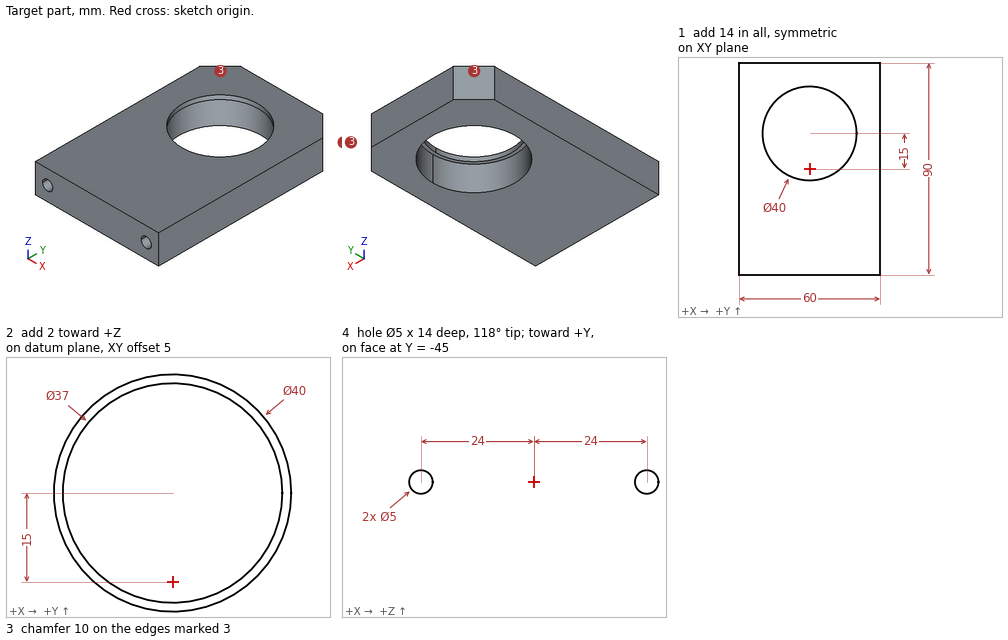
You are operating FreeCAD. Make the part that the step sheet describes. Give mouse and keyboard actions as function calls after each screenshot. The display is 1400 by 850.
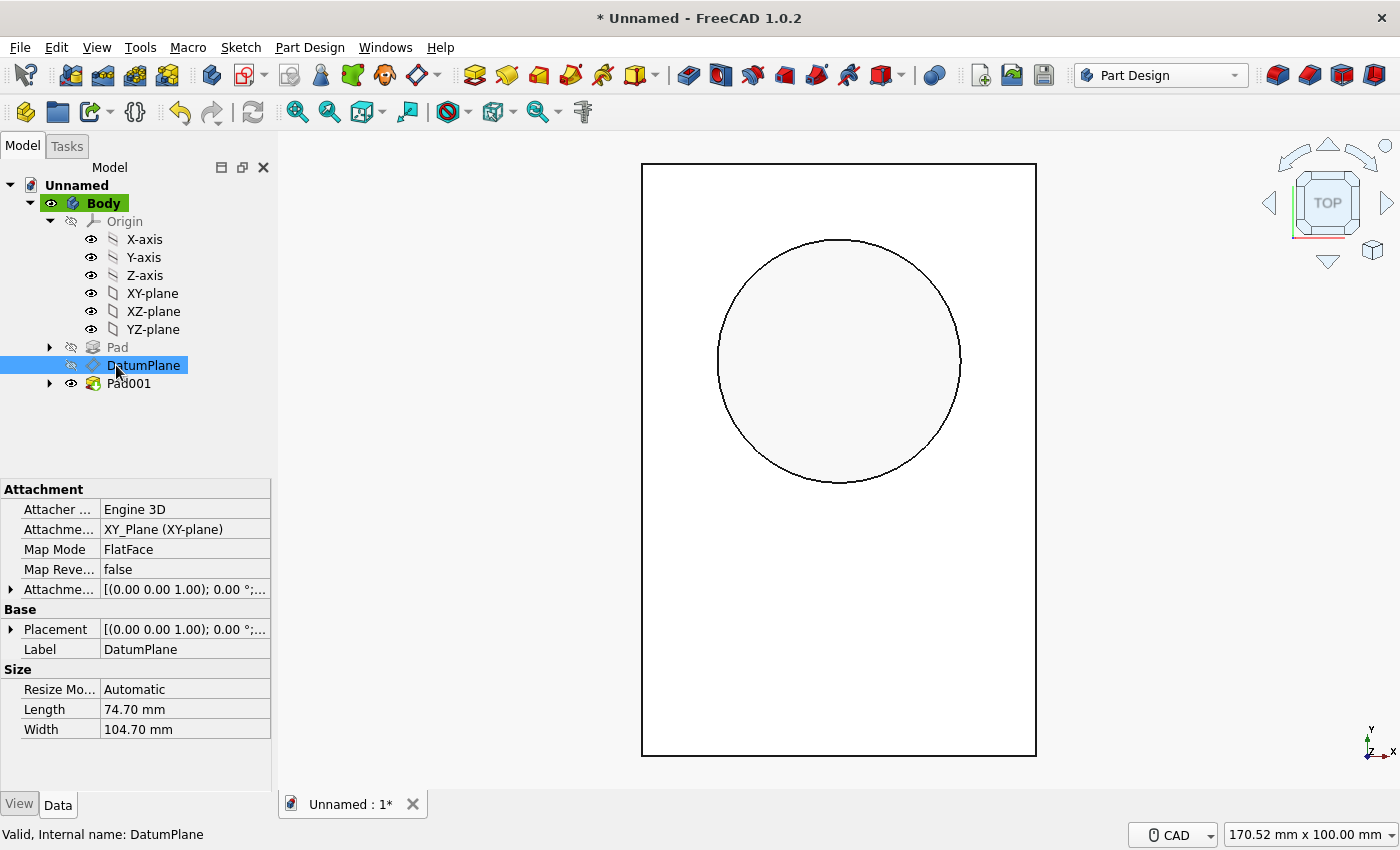
key(1)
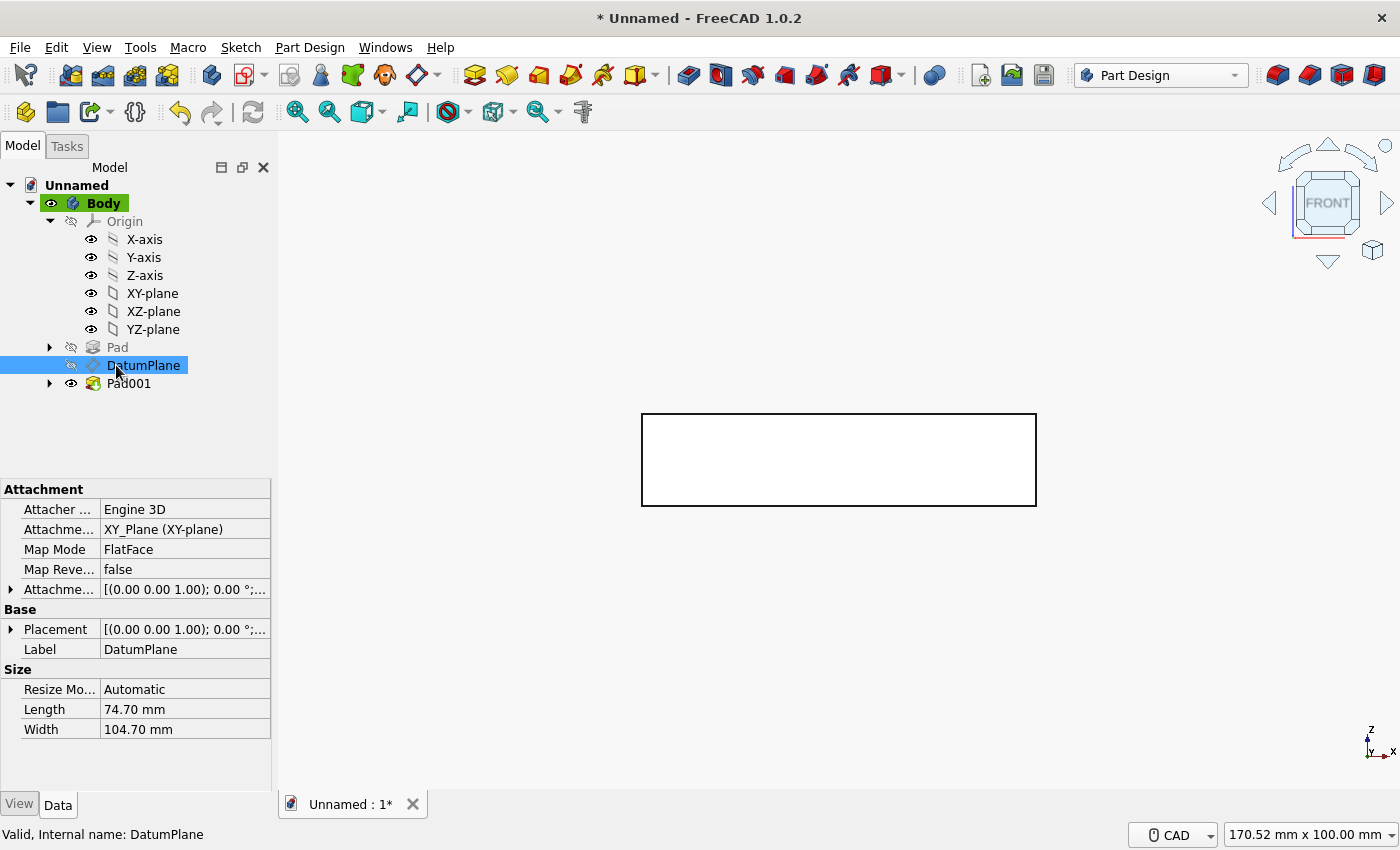
click(298, 112)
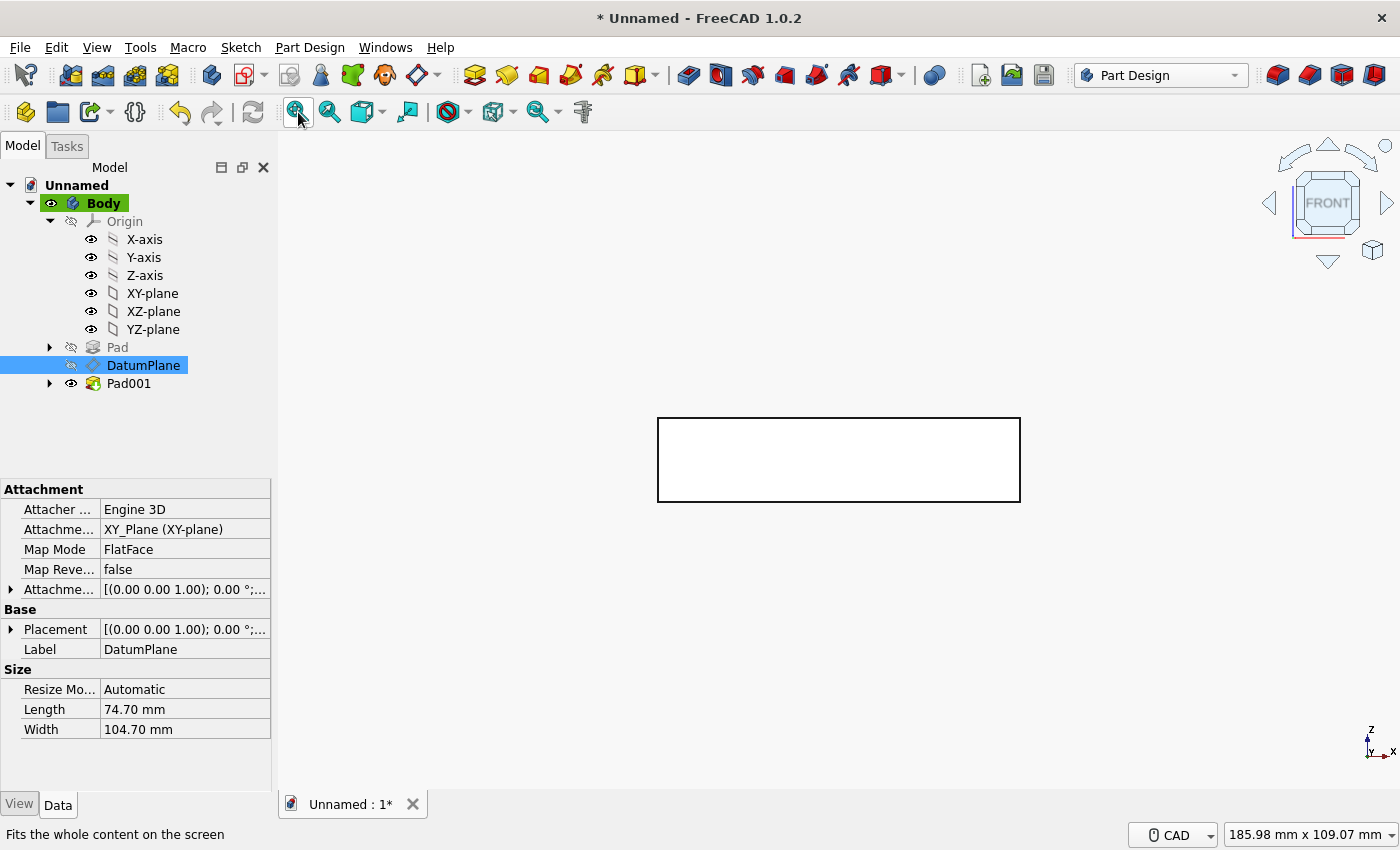
key(3)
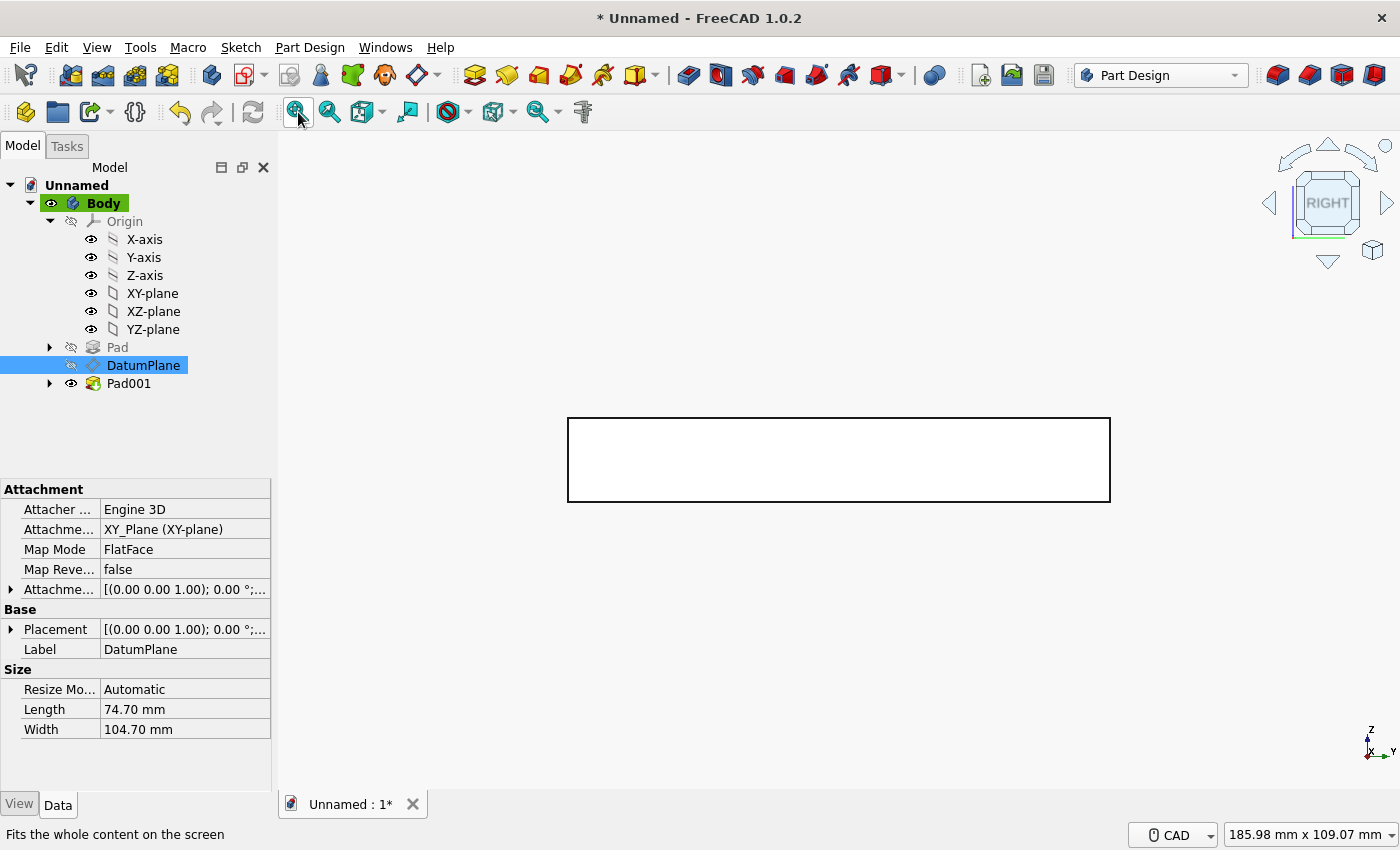
click(1110, 459)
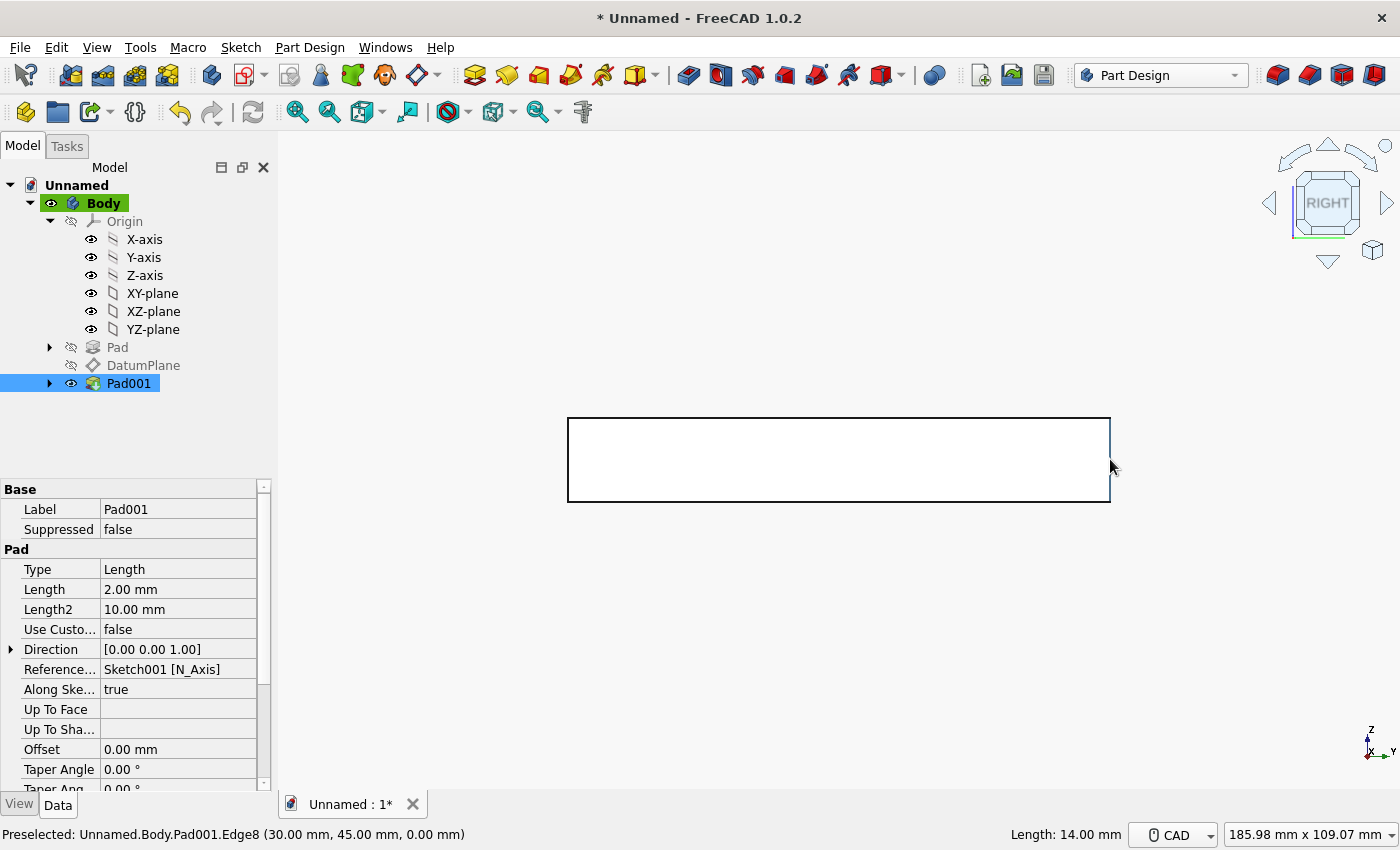
key(5)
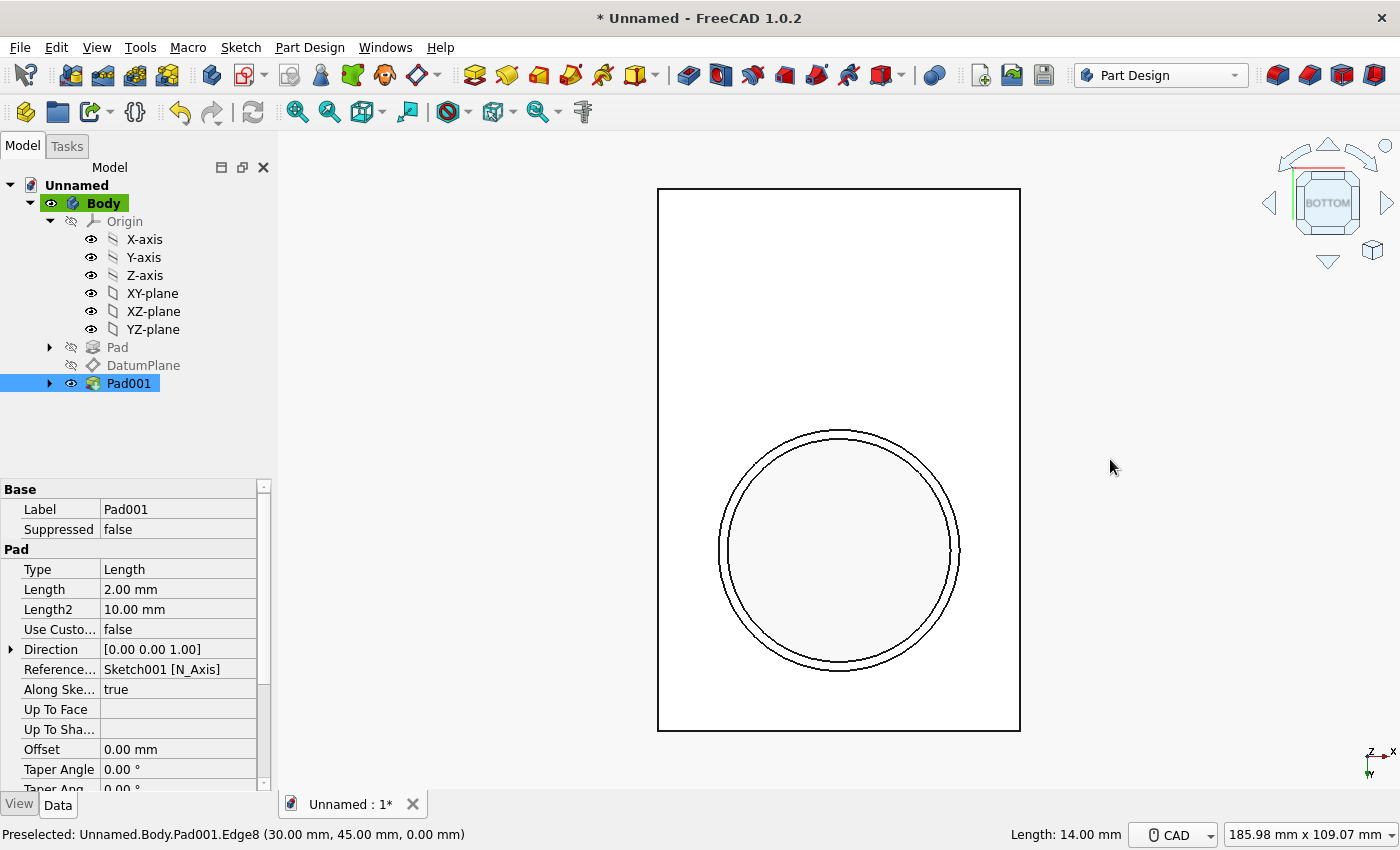
key(4)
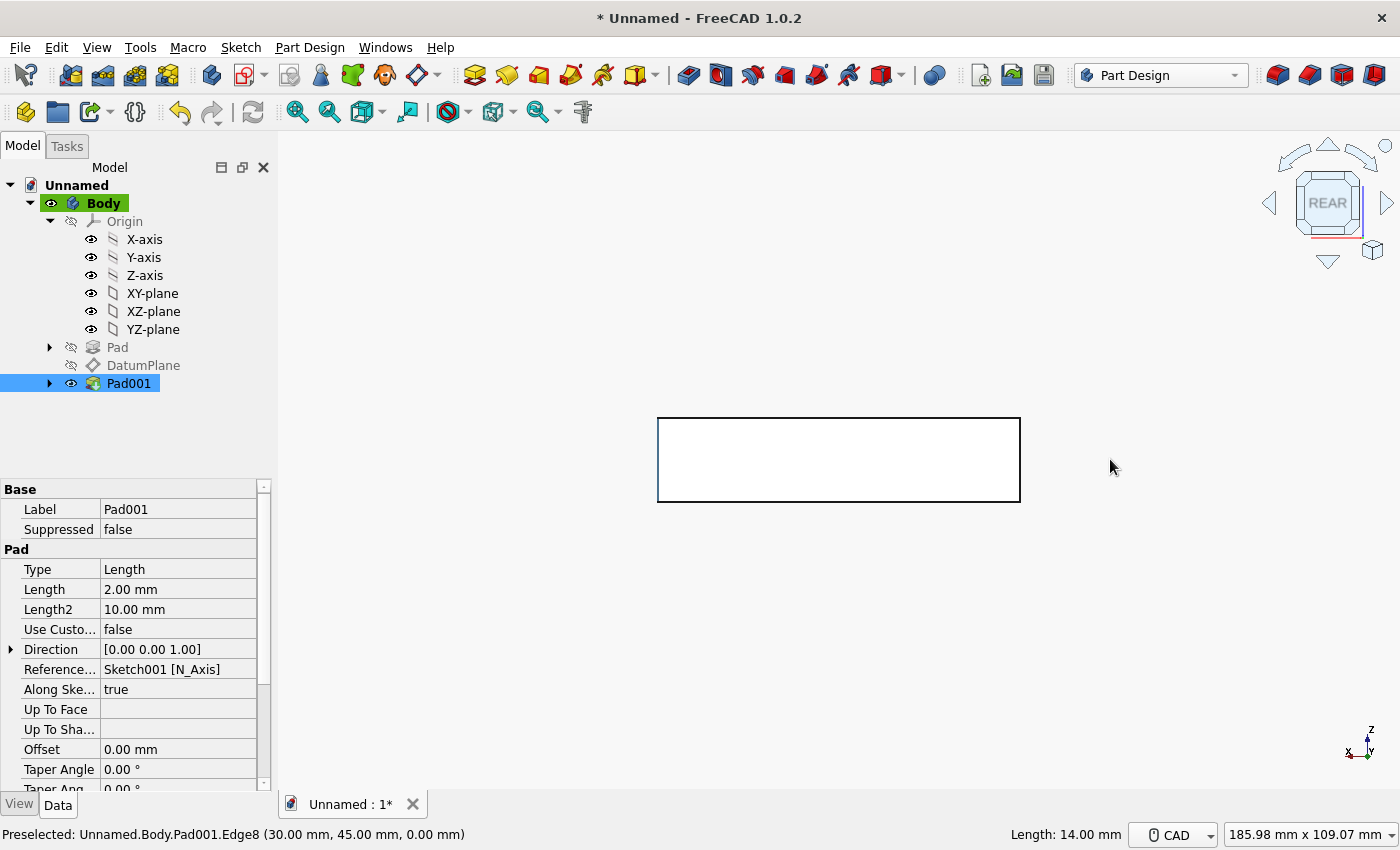
click(298, 112)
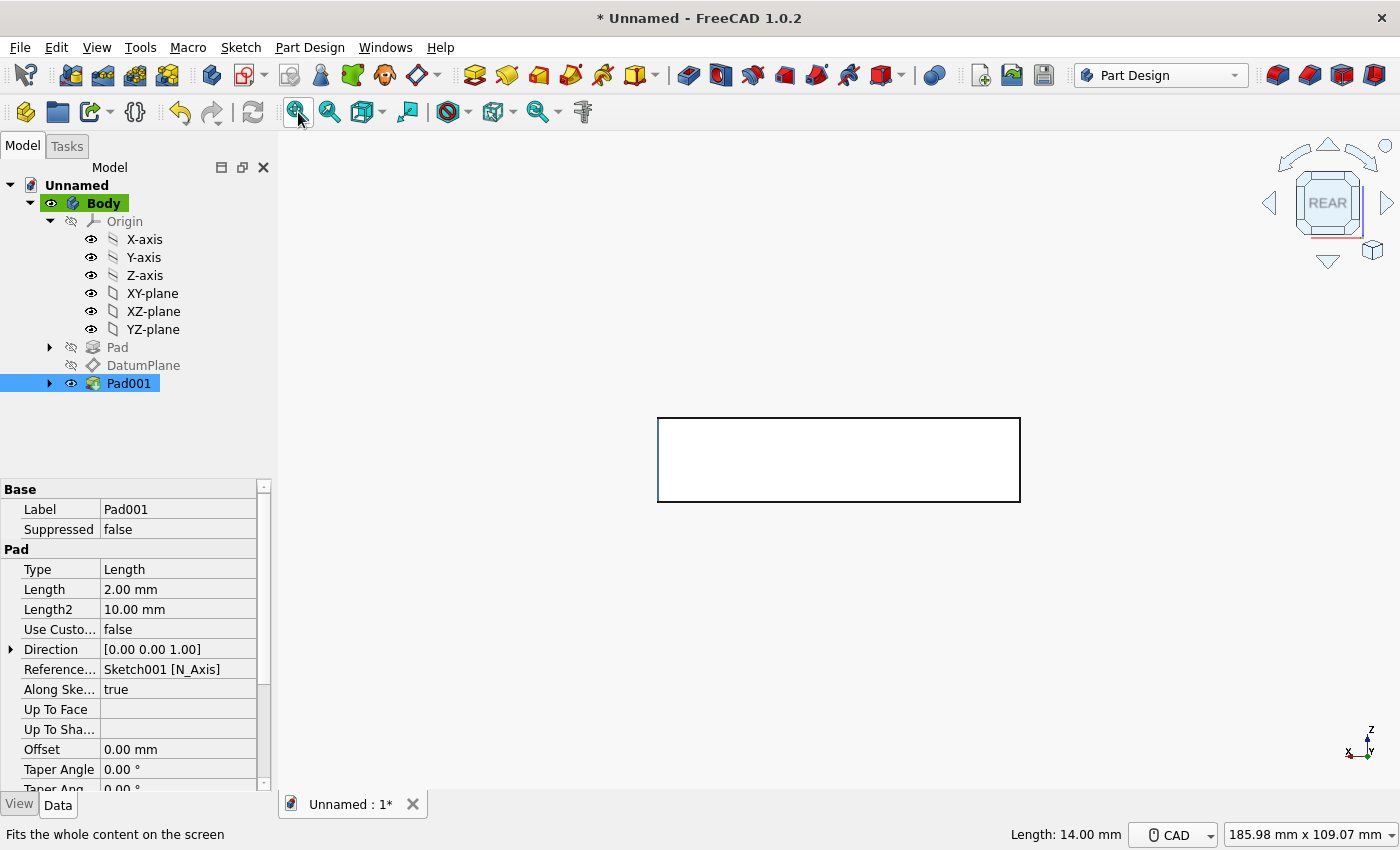
click(1020, 459, ctrl)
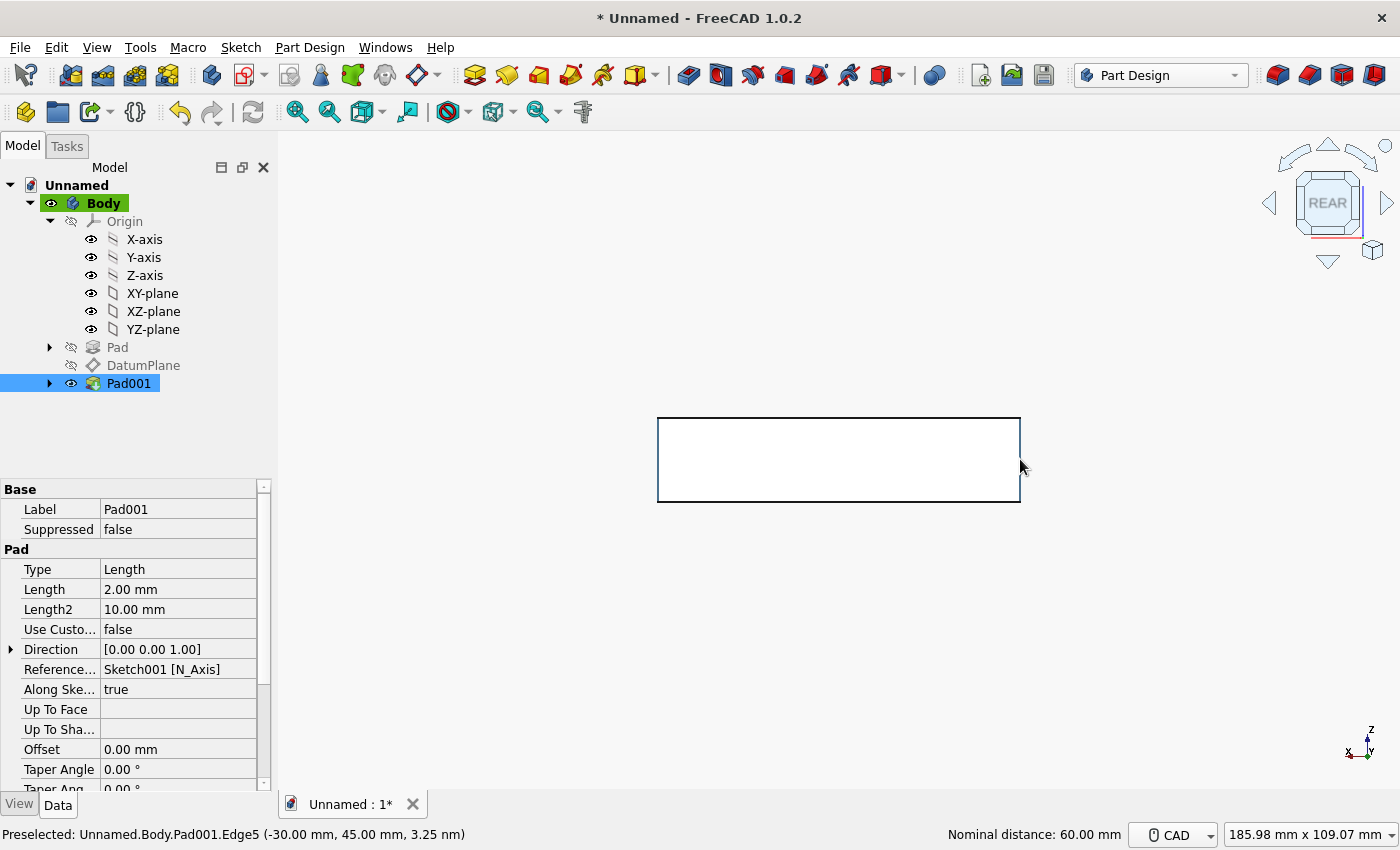
click(1310, 76)